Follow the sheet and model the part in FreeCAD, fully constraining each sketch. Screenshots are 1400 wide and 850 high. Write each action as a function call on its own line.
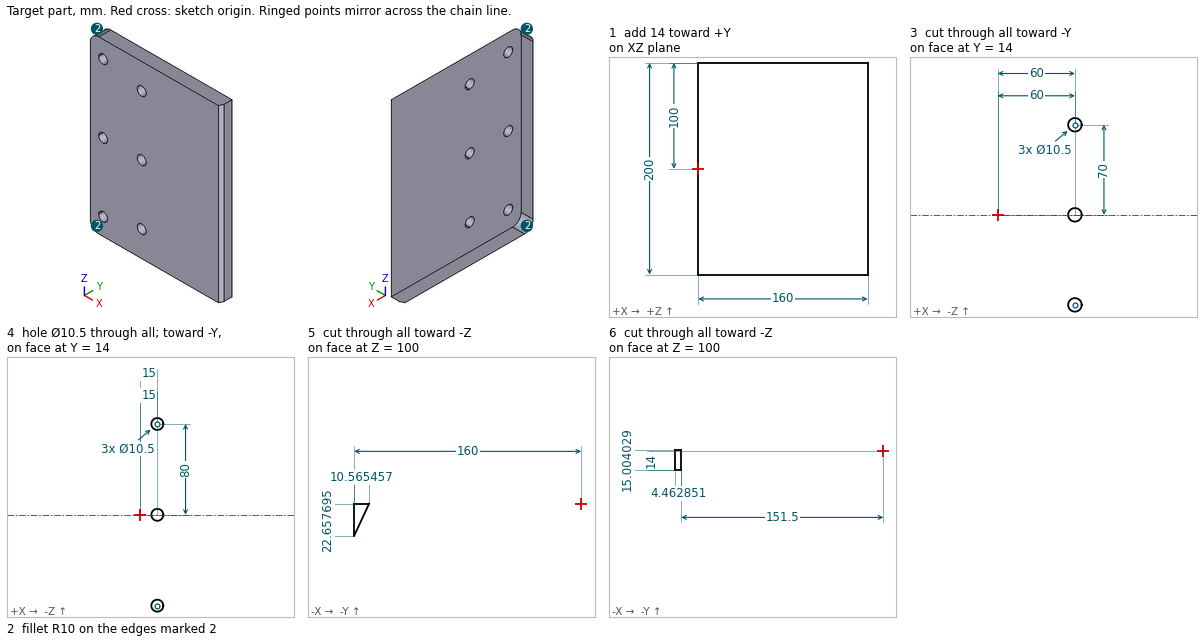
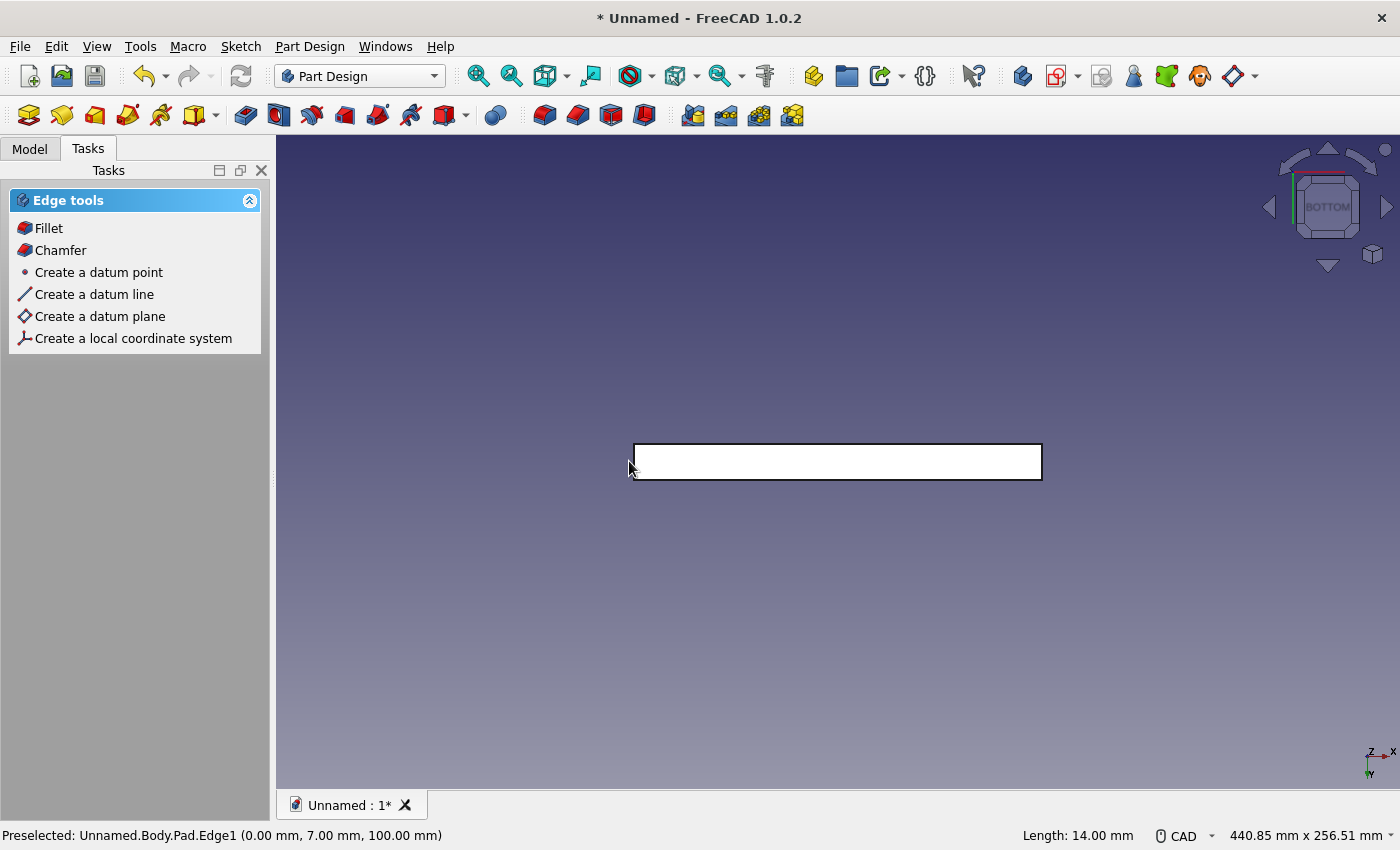
click(479, 76)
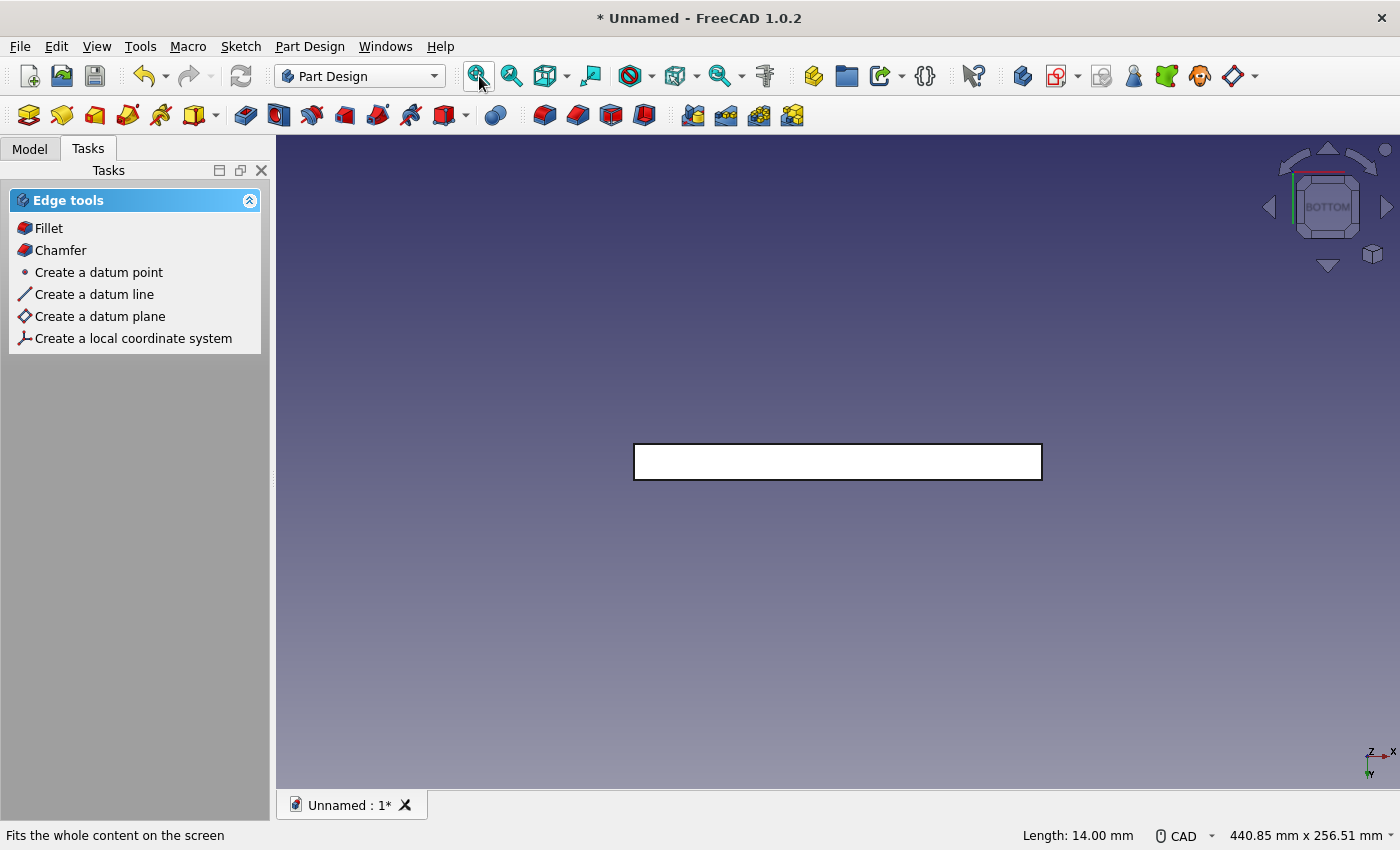
click(634, 461, ctrl)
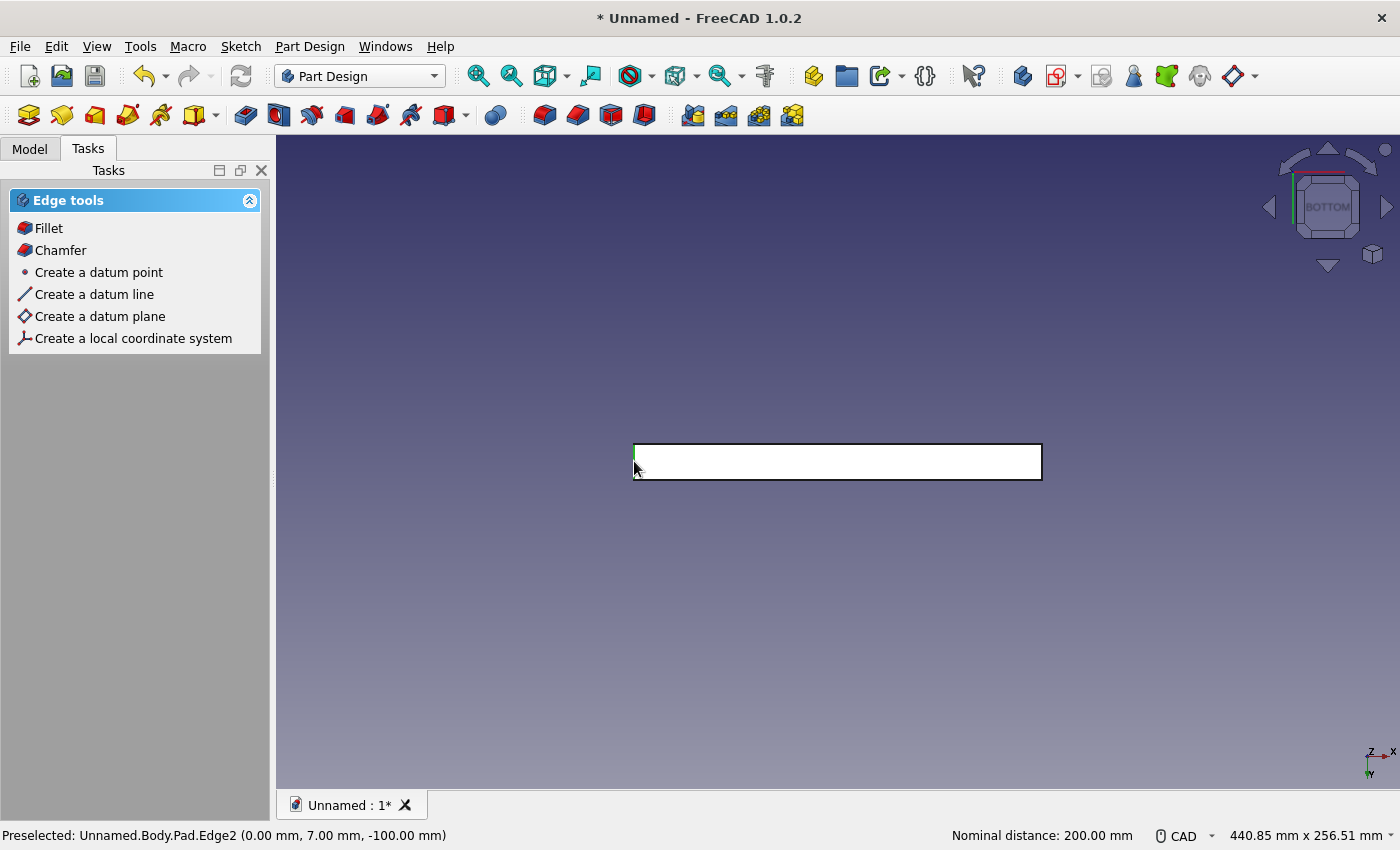
click(545, 116)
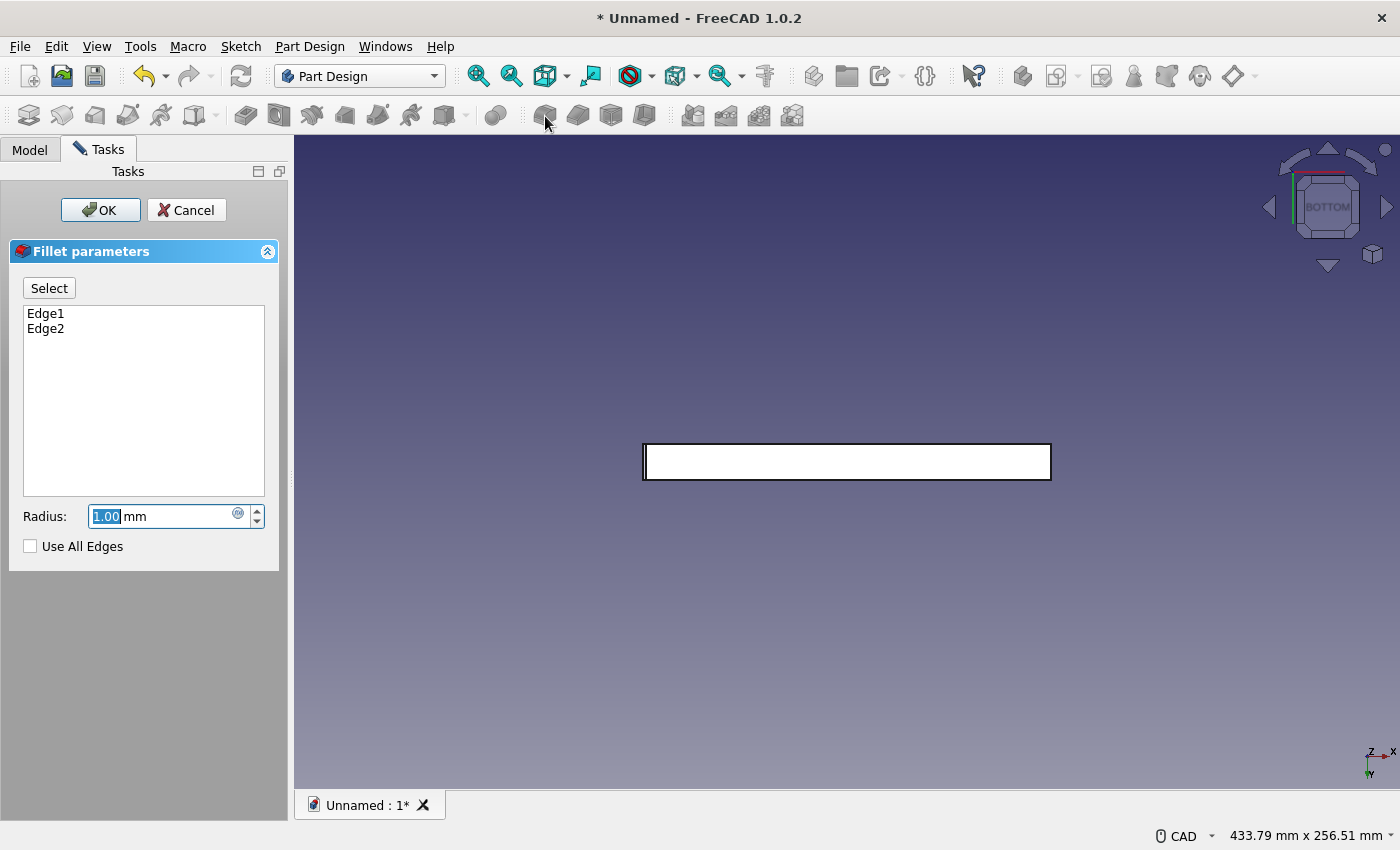
text(10)
key(Tab)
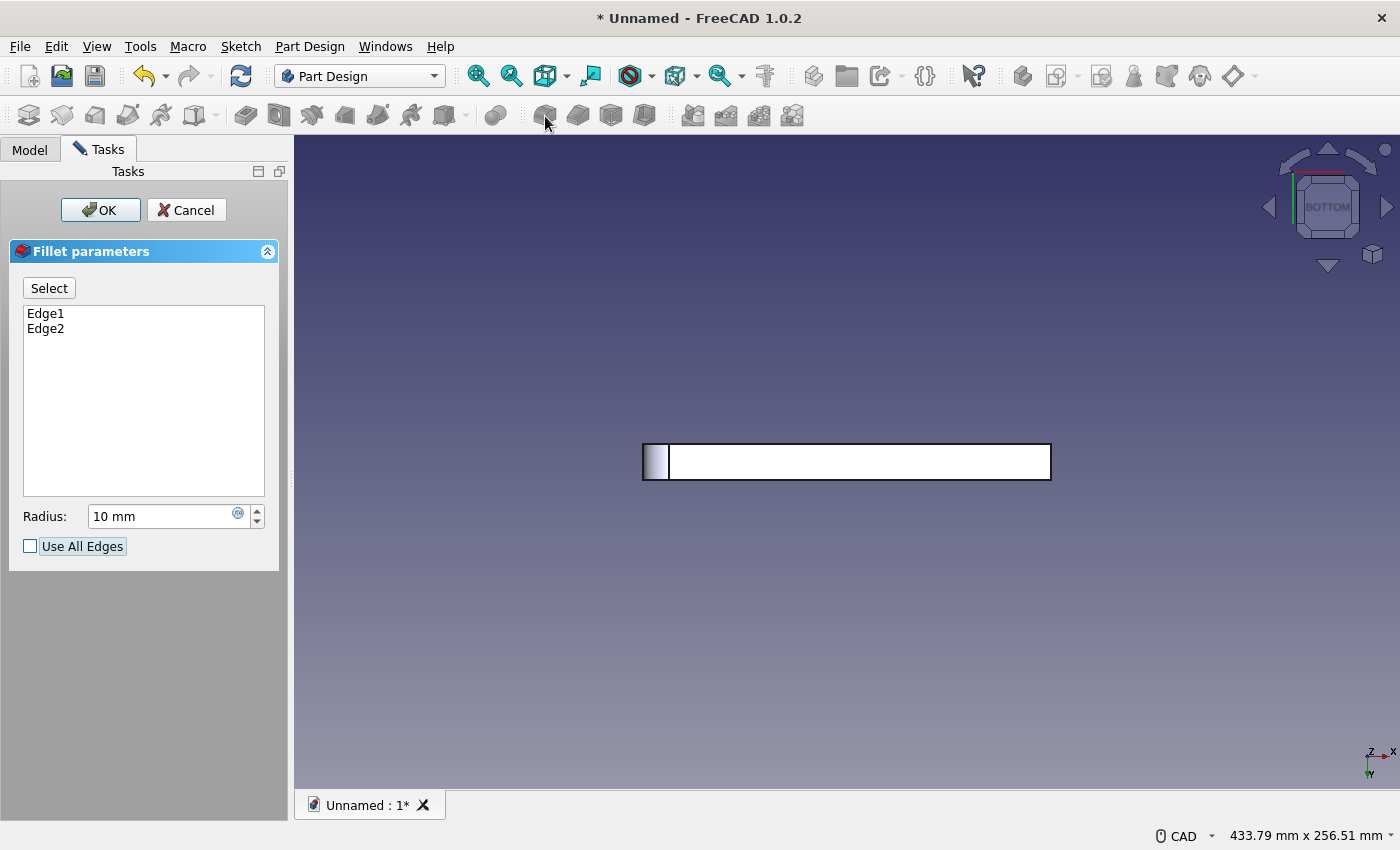
click(101, 210)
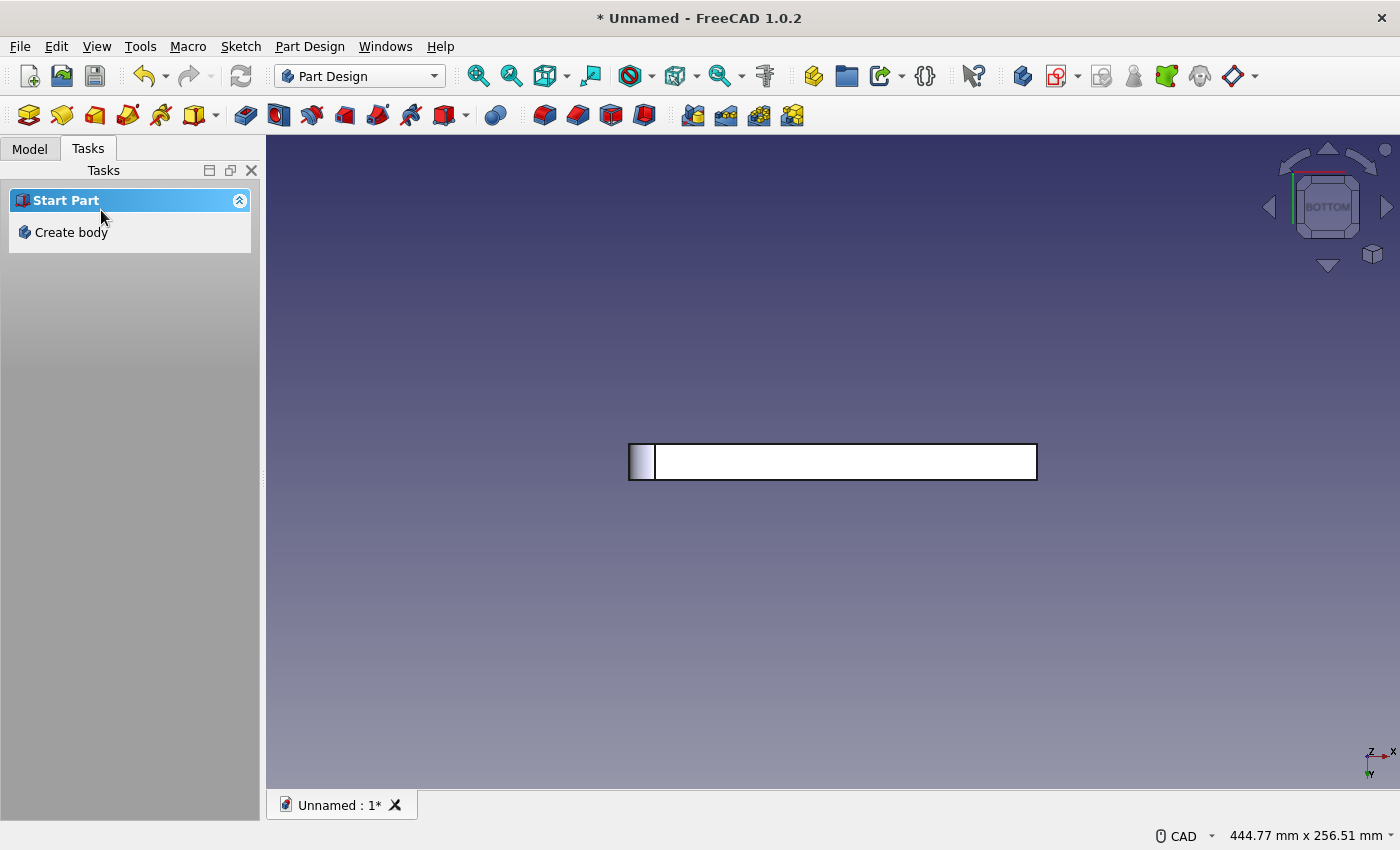
click(479, 76)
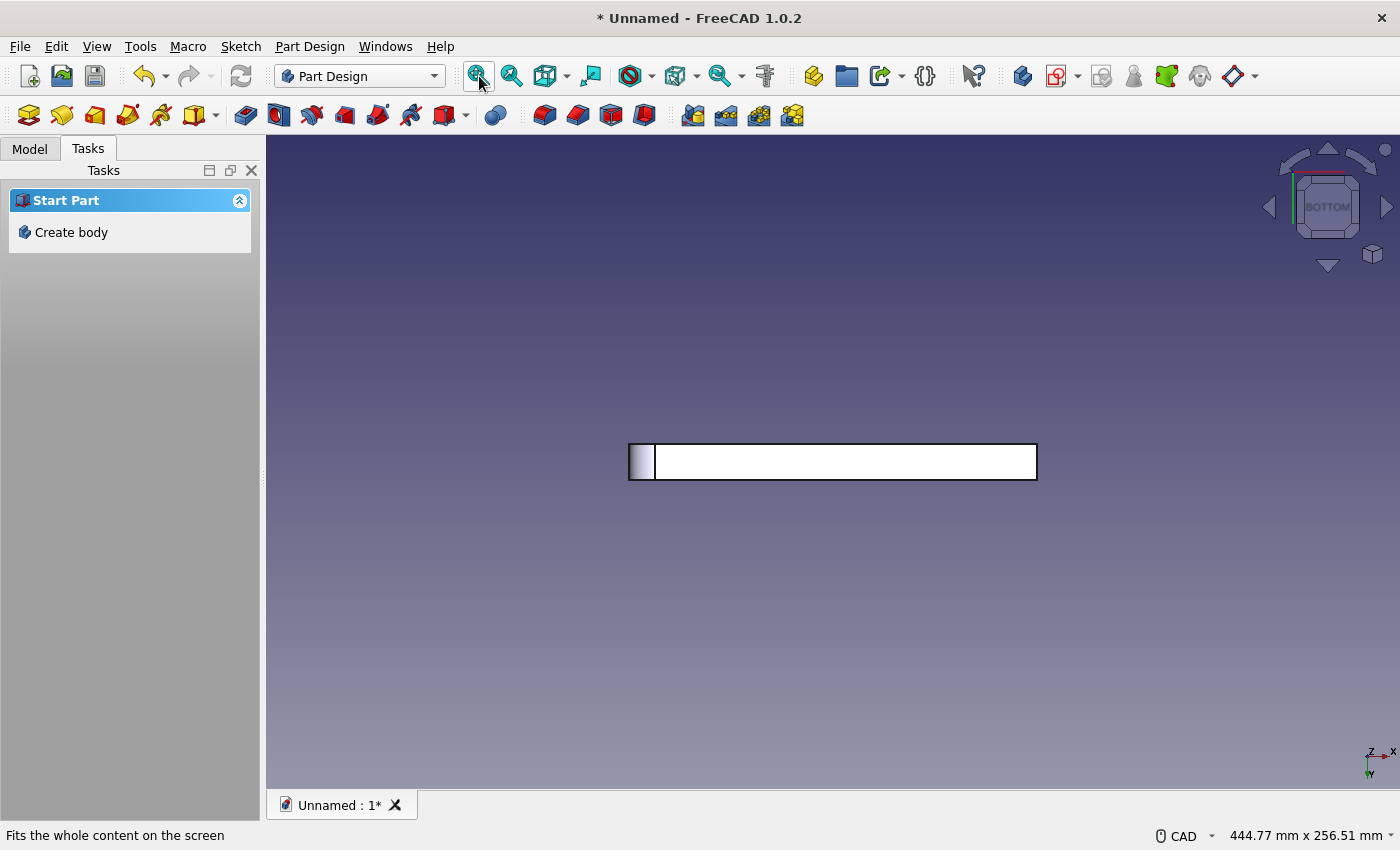
key(4)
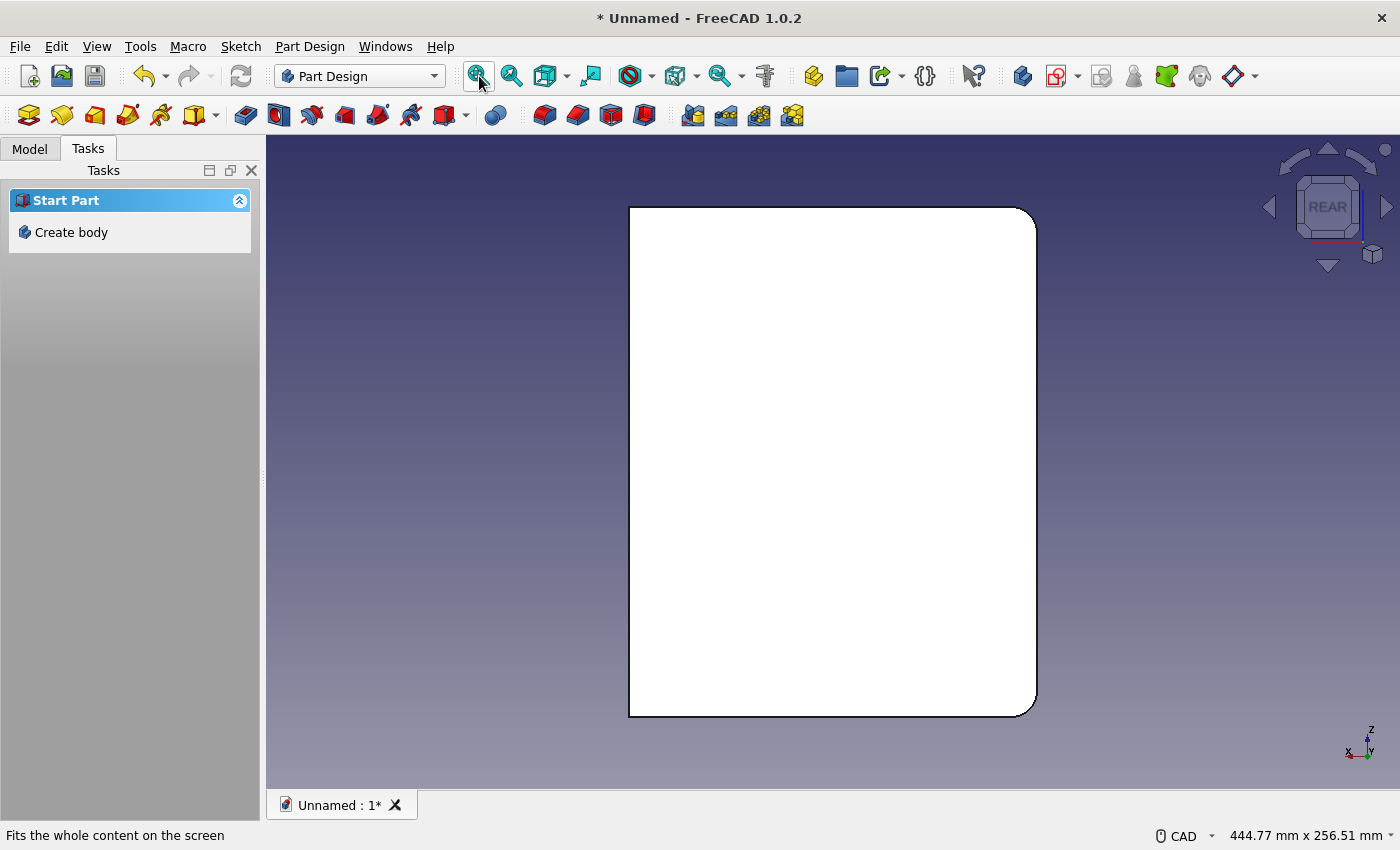
click(833, 461)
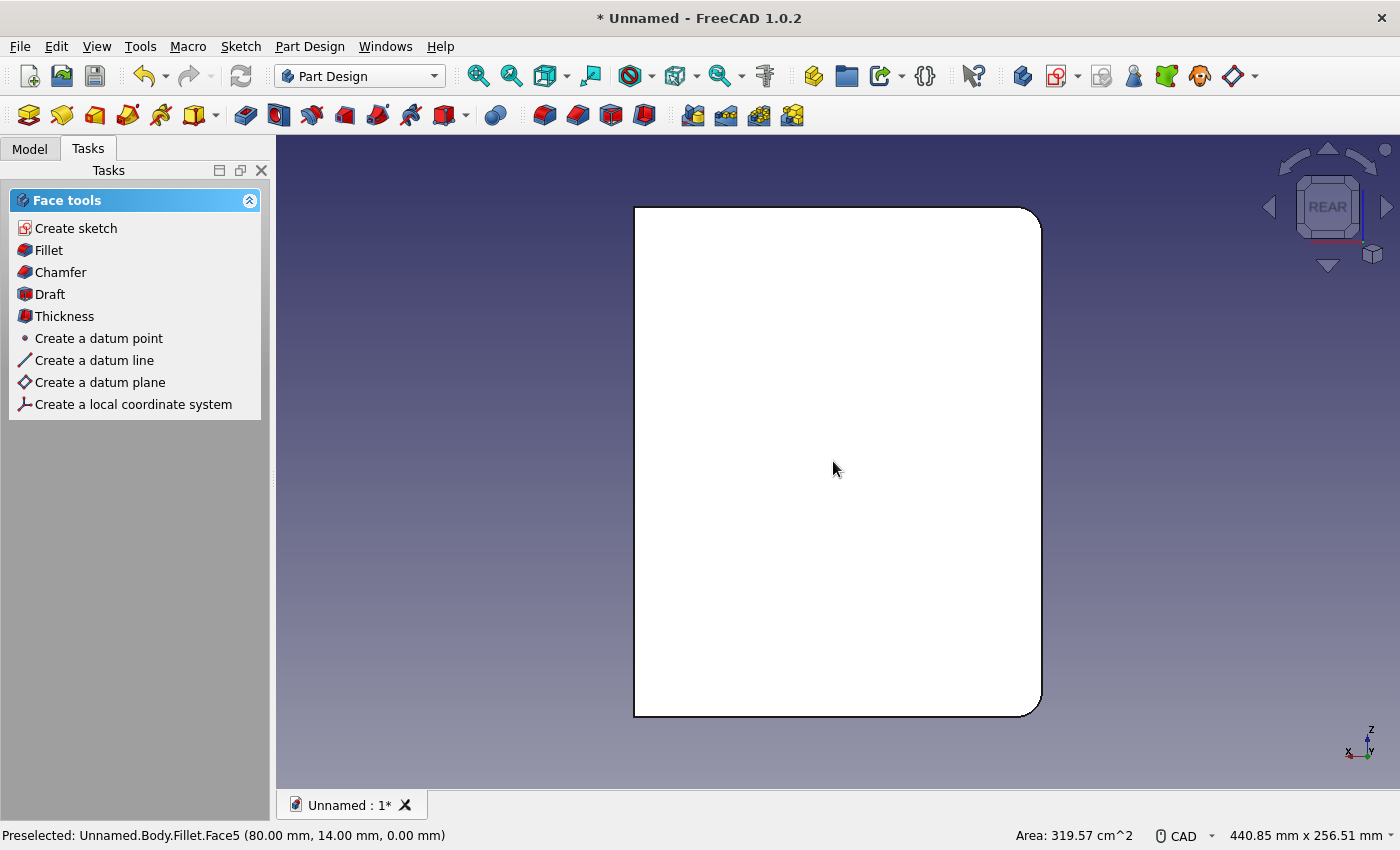
click(1056, 76)